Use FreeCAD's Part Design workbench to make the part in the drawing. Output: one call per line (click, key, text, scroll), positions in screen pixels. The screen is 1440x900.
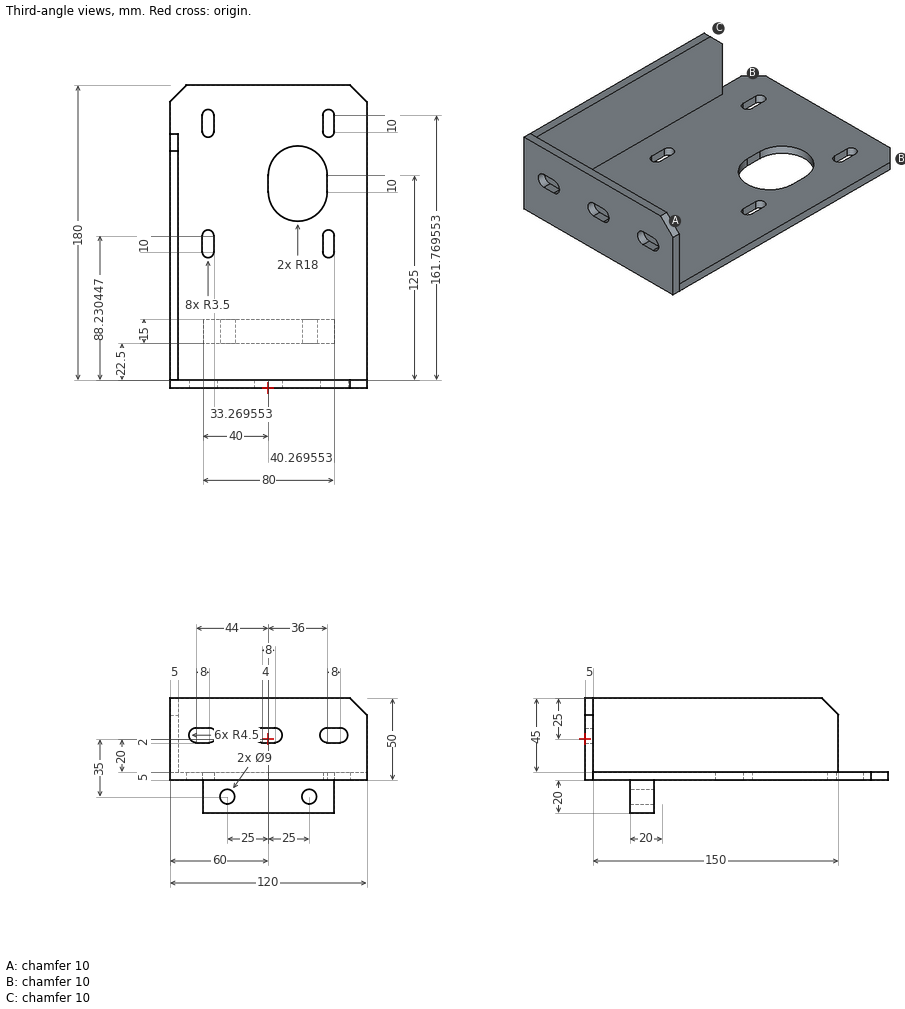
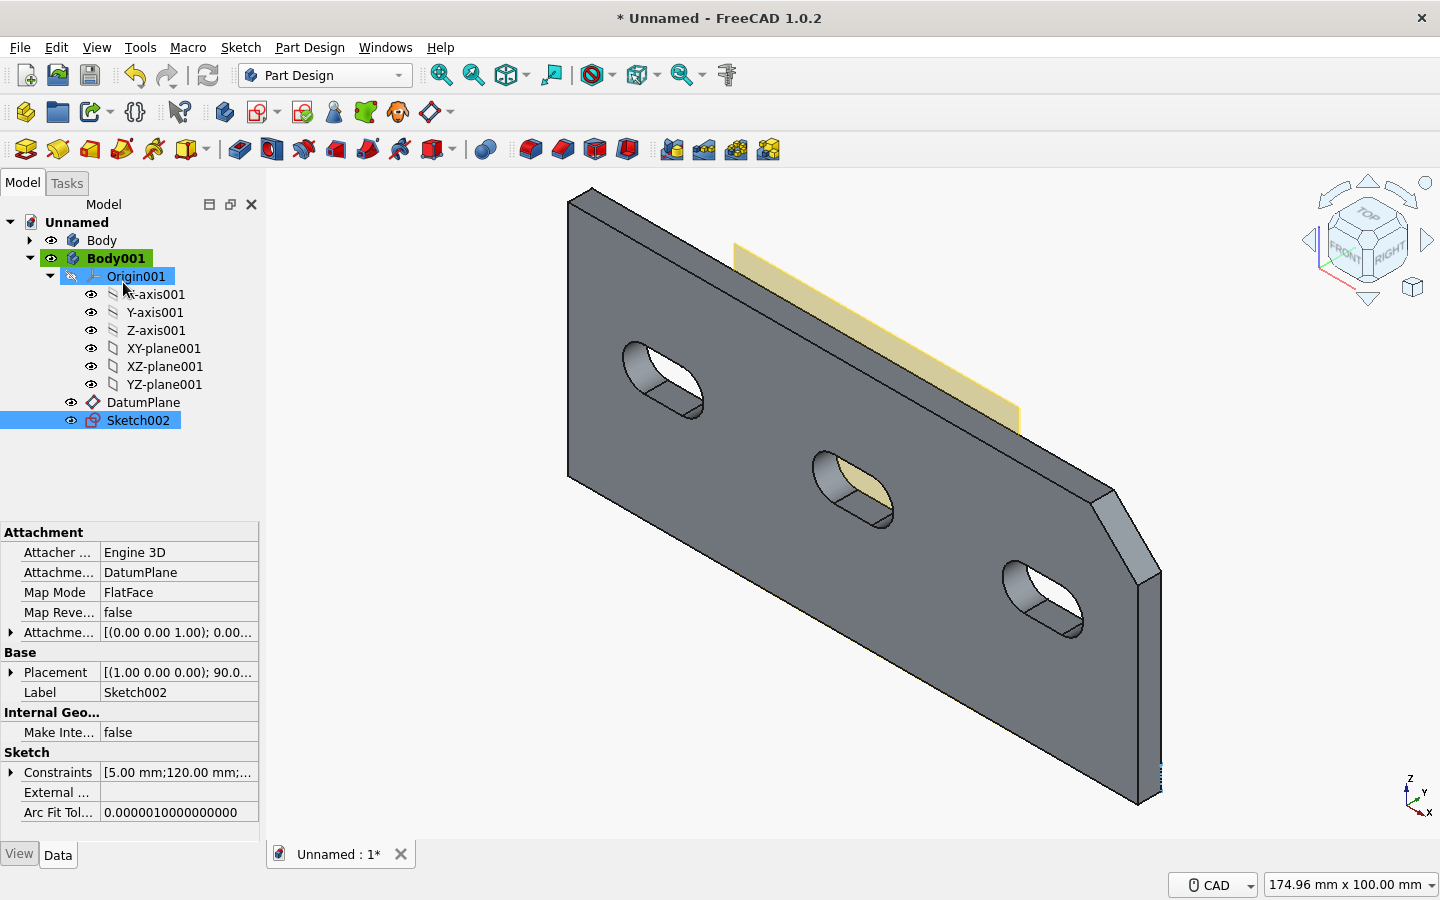
click(26, 150)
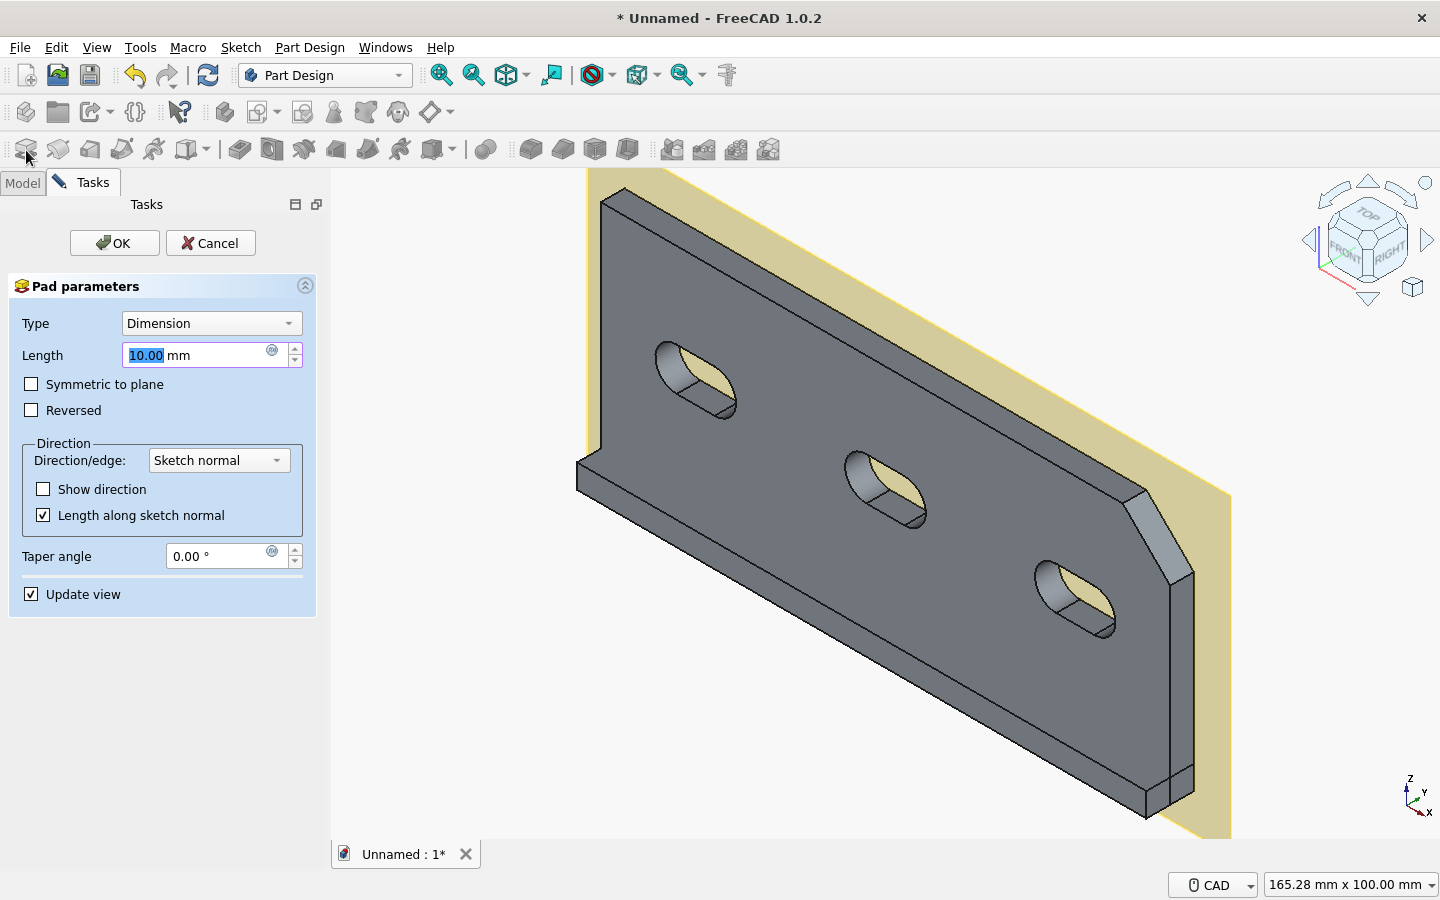
text(180)
key(Tab)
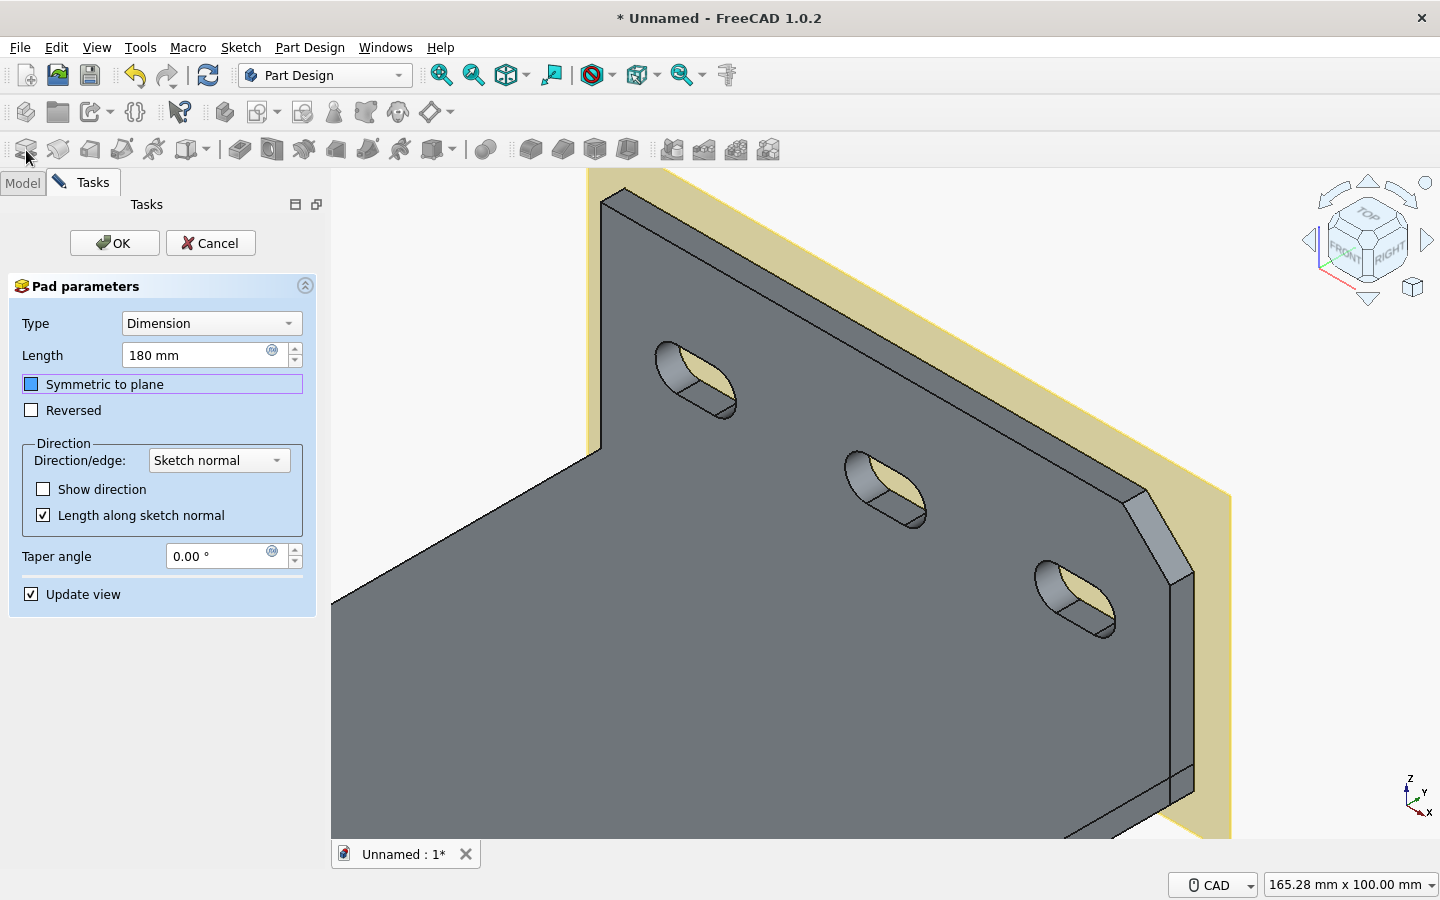
click(30, 410)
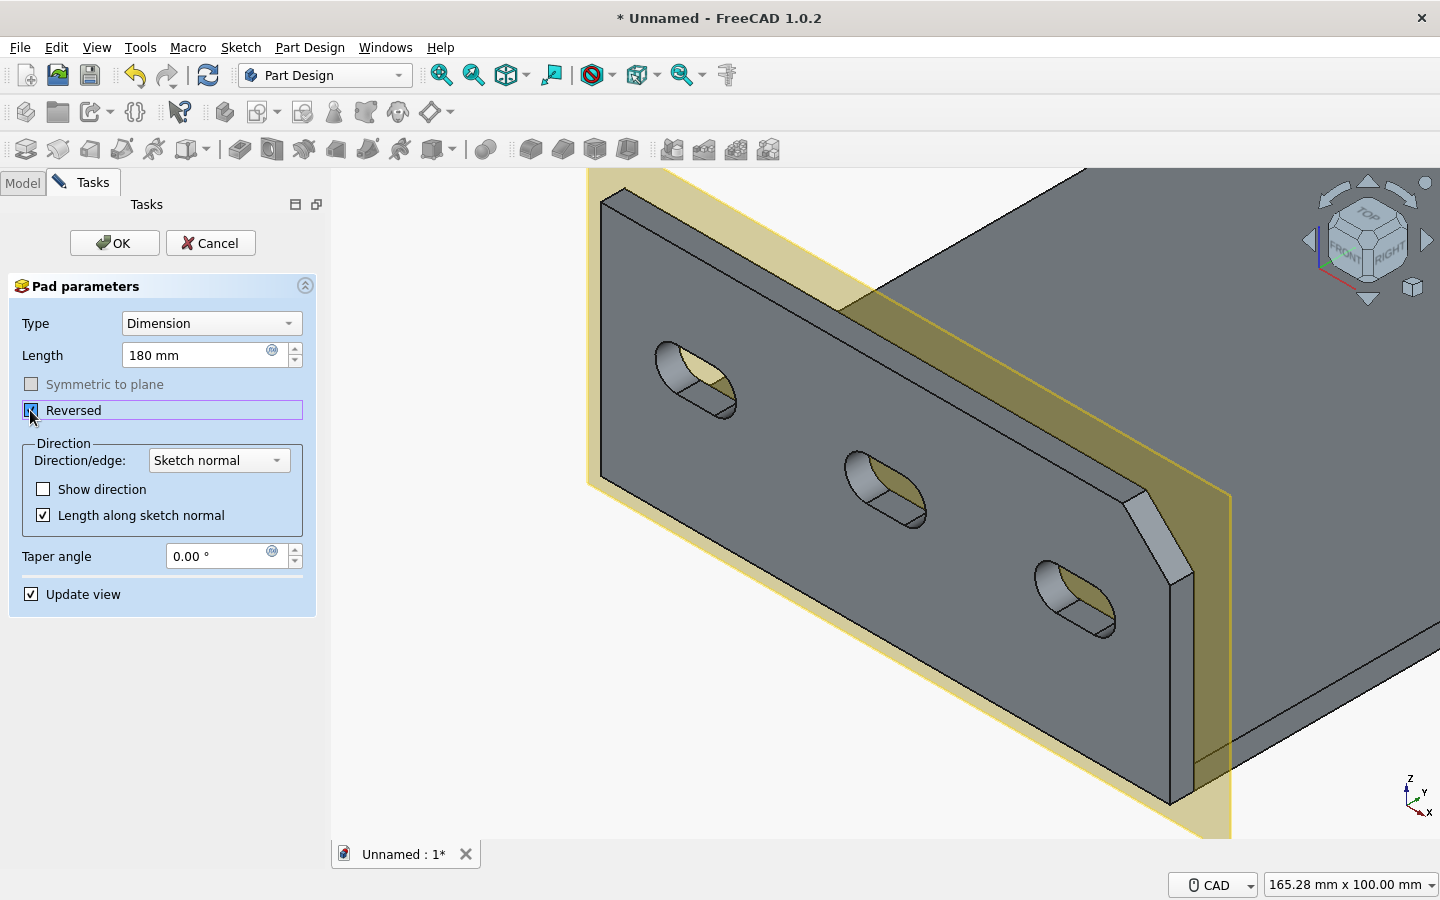
click(115, 243)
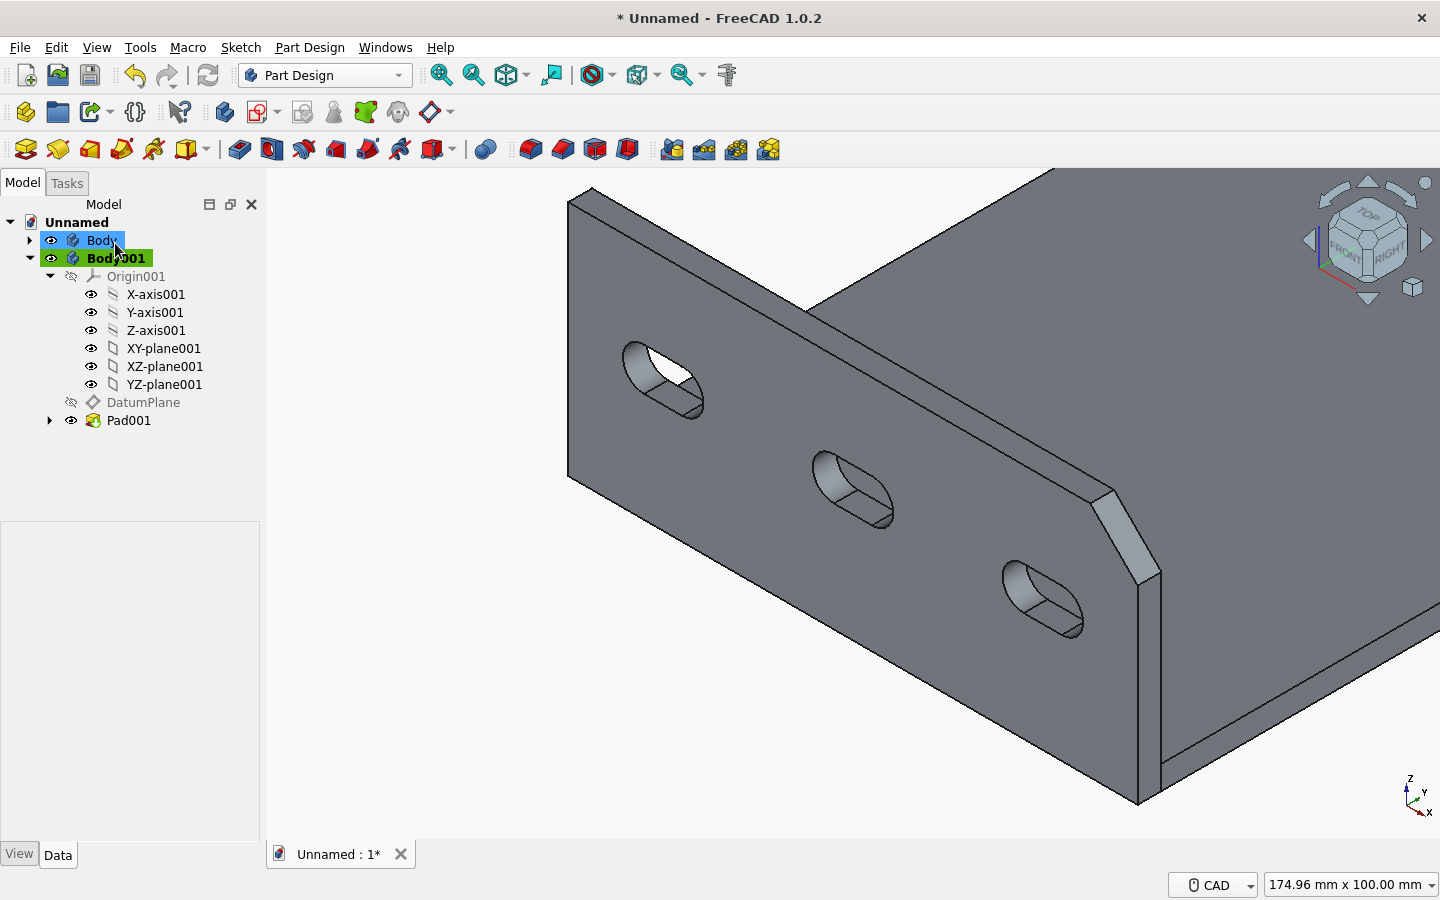
key(v)
key(f)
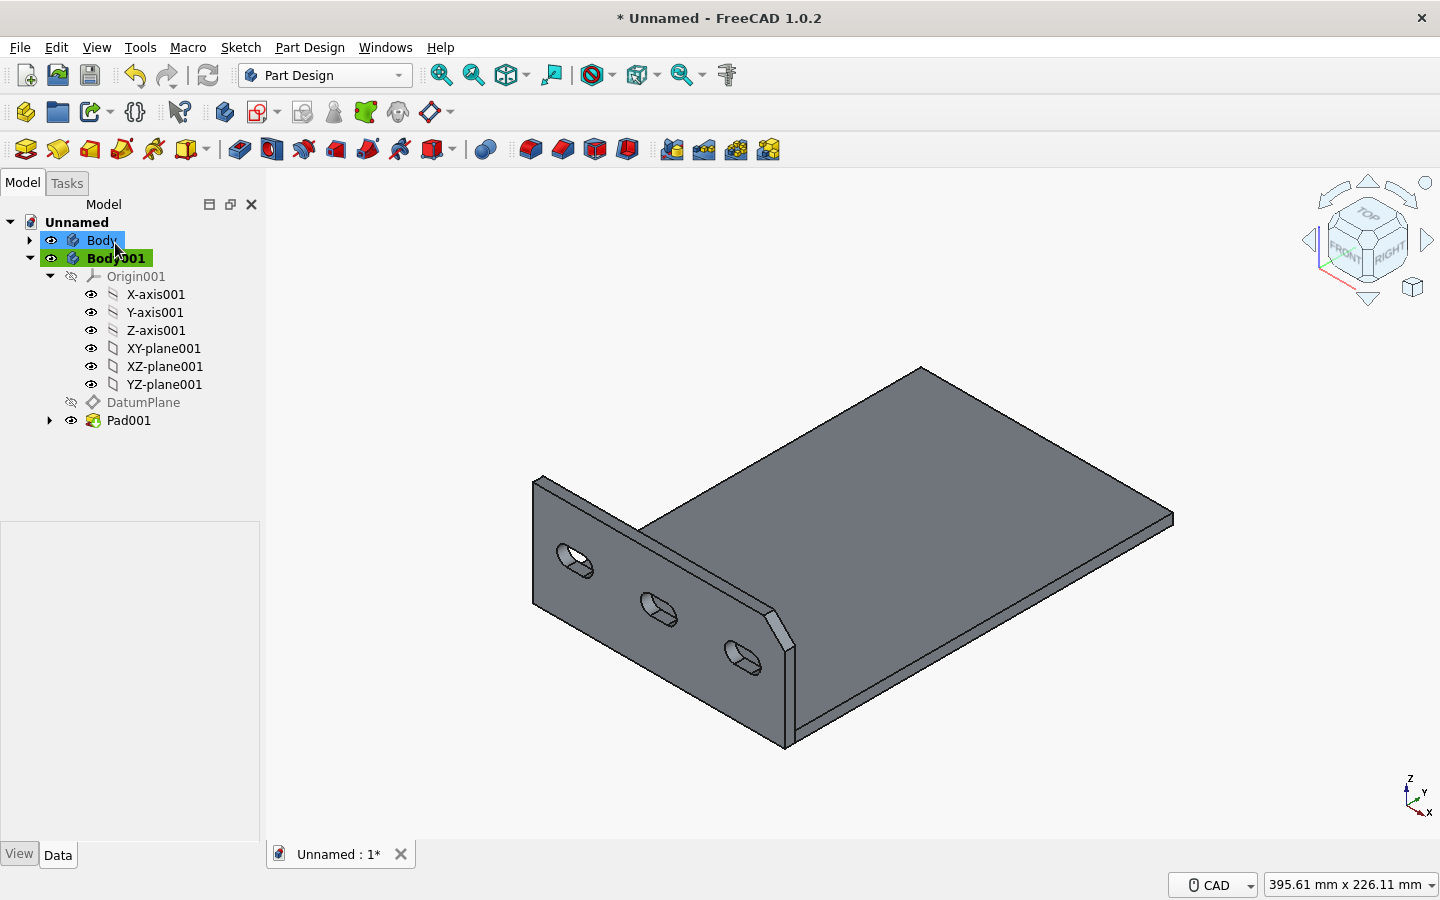
click(912, 517)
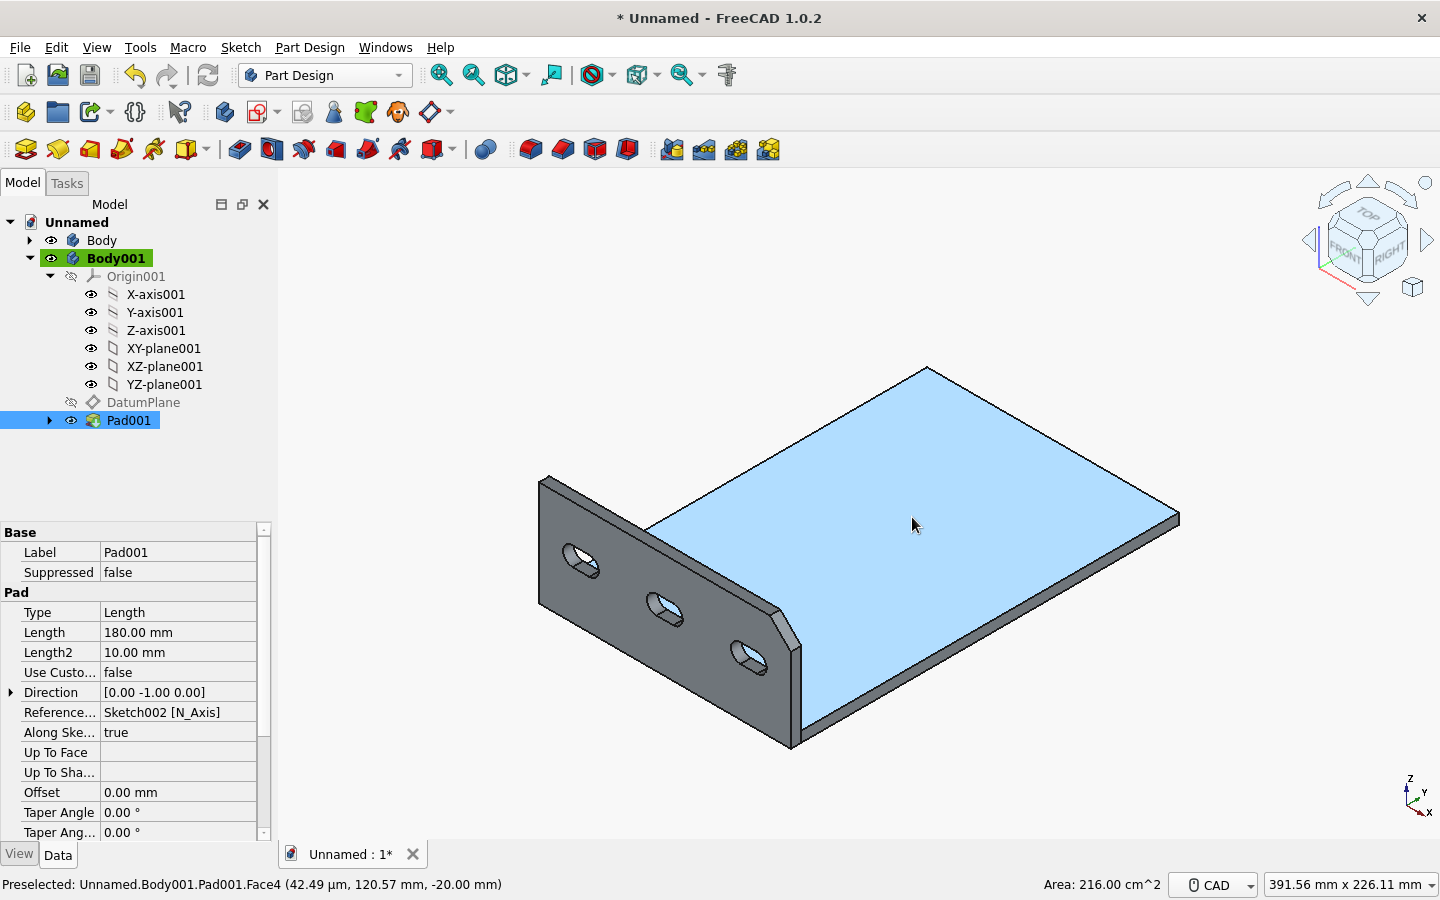
click(258, 112)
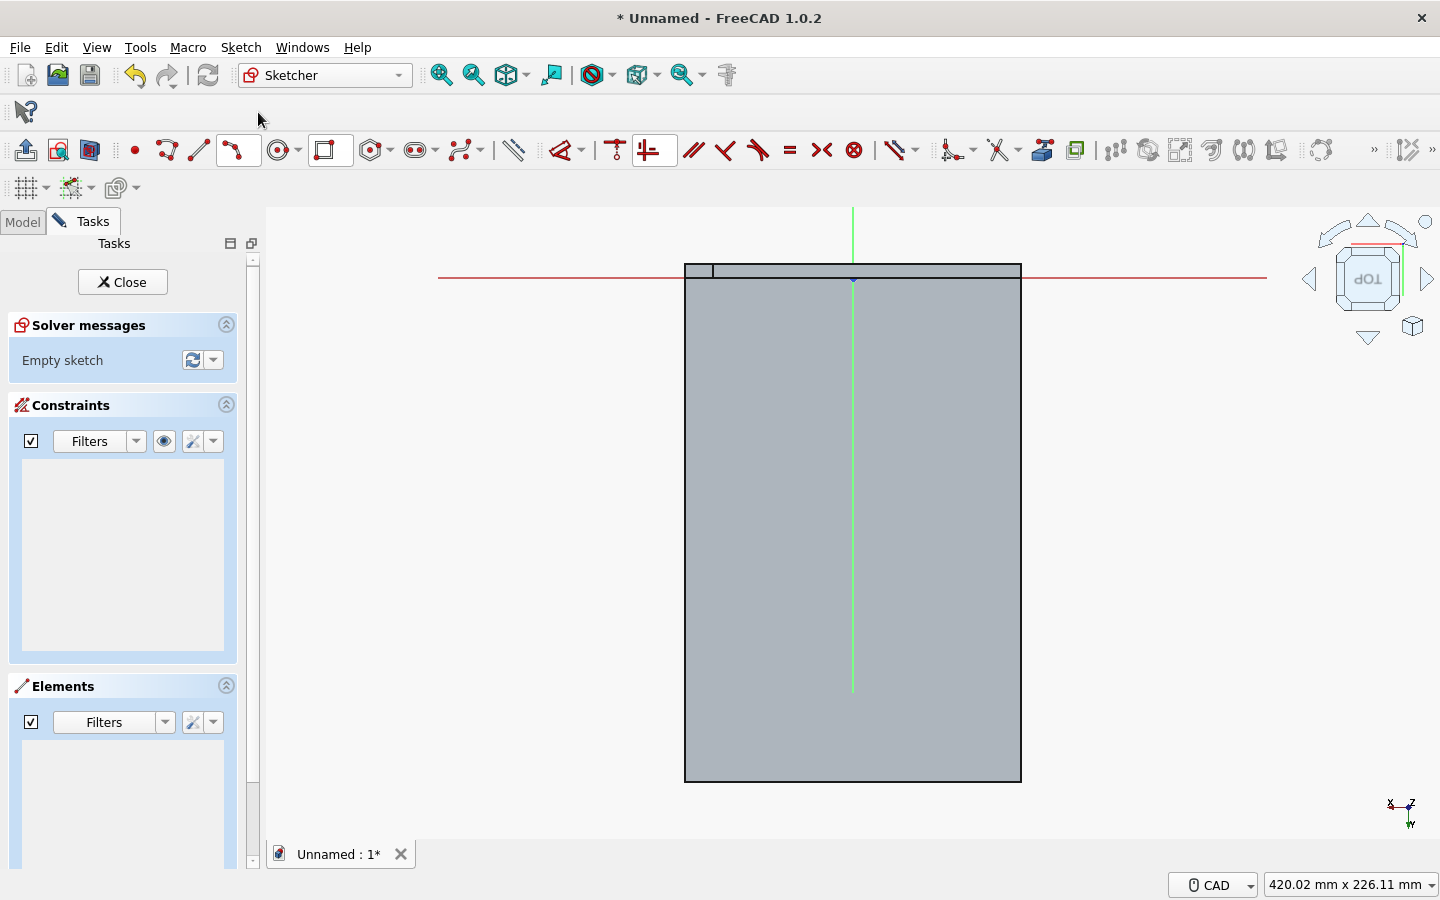
click(416, 150)